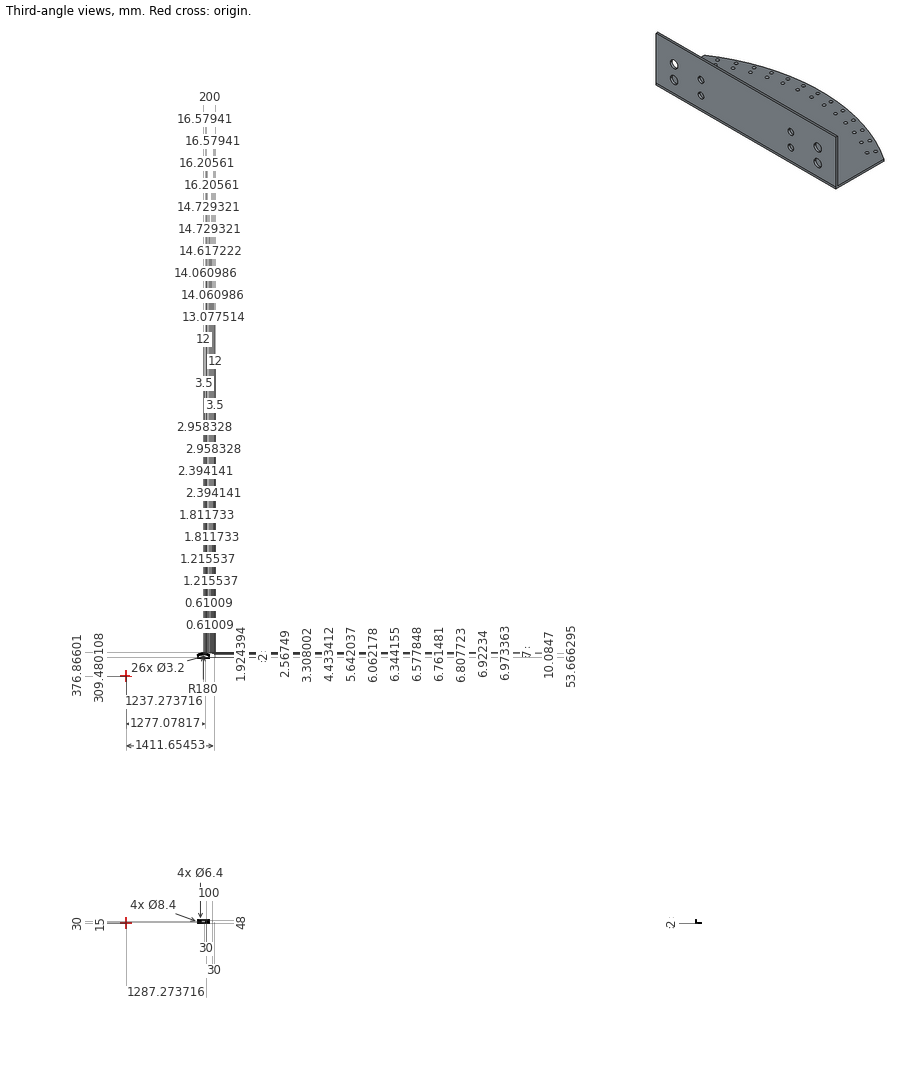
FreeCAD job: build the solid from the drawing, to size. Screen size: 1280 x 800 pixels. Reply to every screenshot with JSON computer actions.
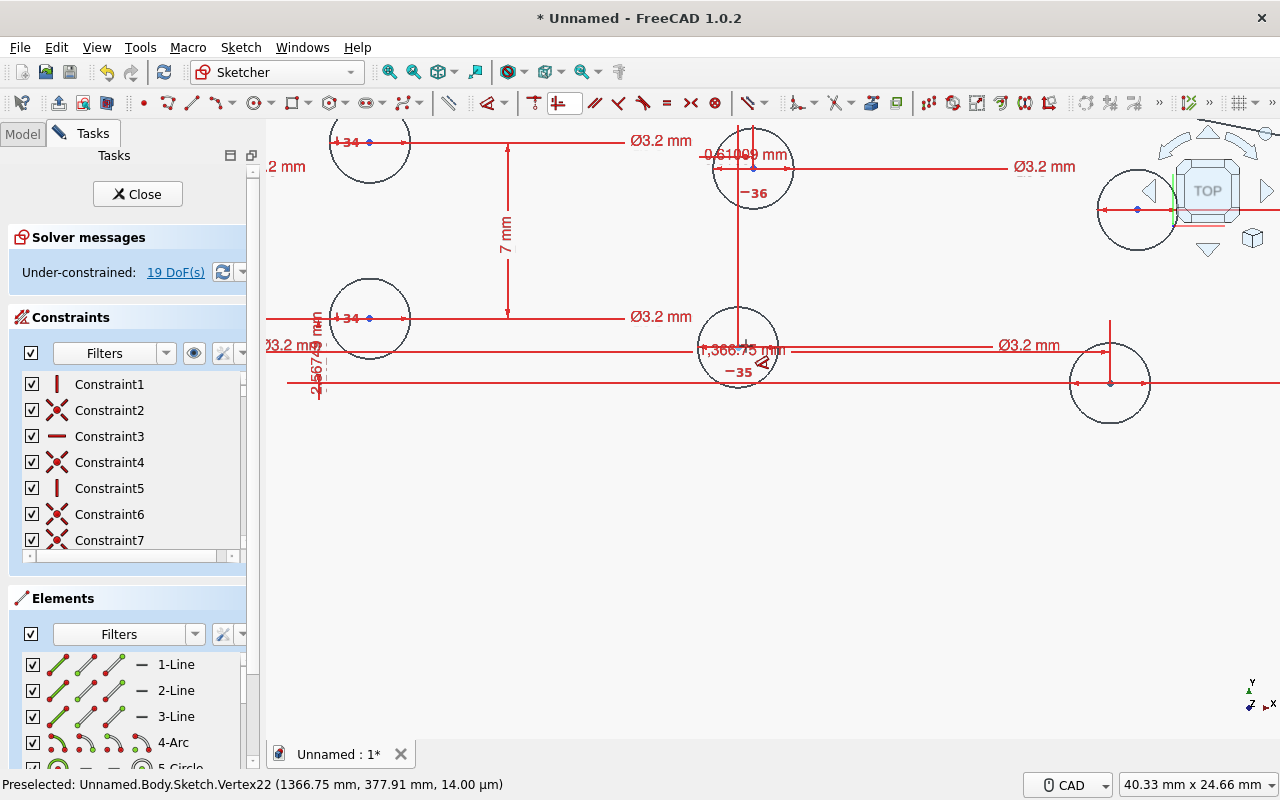
{"action": "left_click", "coordinate": [738, 347]}
{"action": "left_click", "coordinate": [680, 365]}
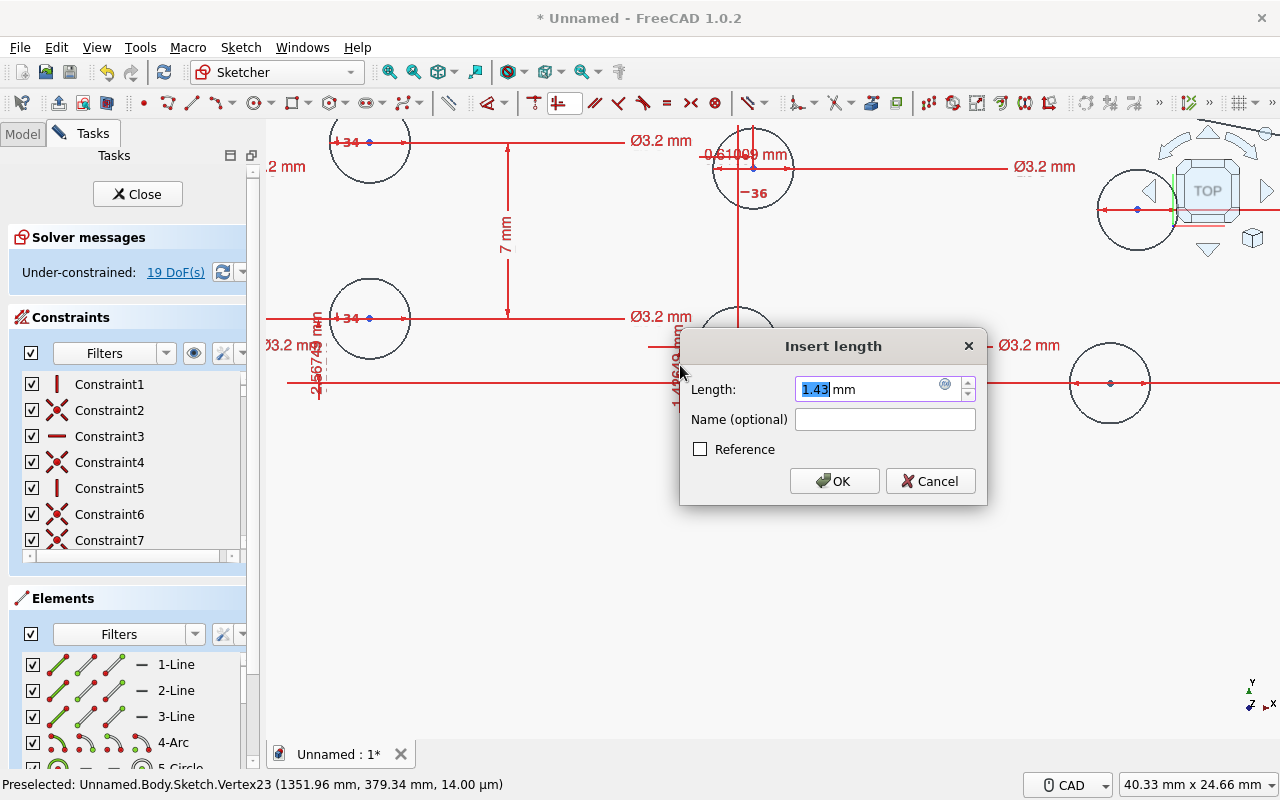
{"action": "type", "text": "1.924394"}
{"action": "key", "text": "Return"}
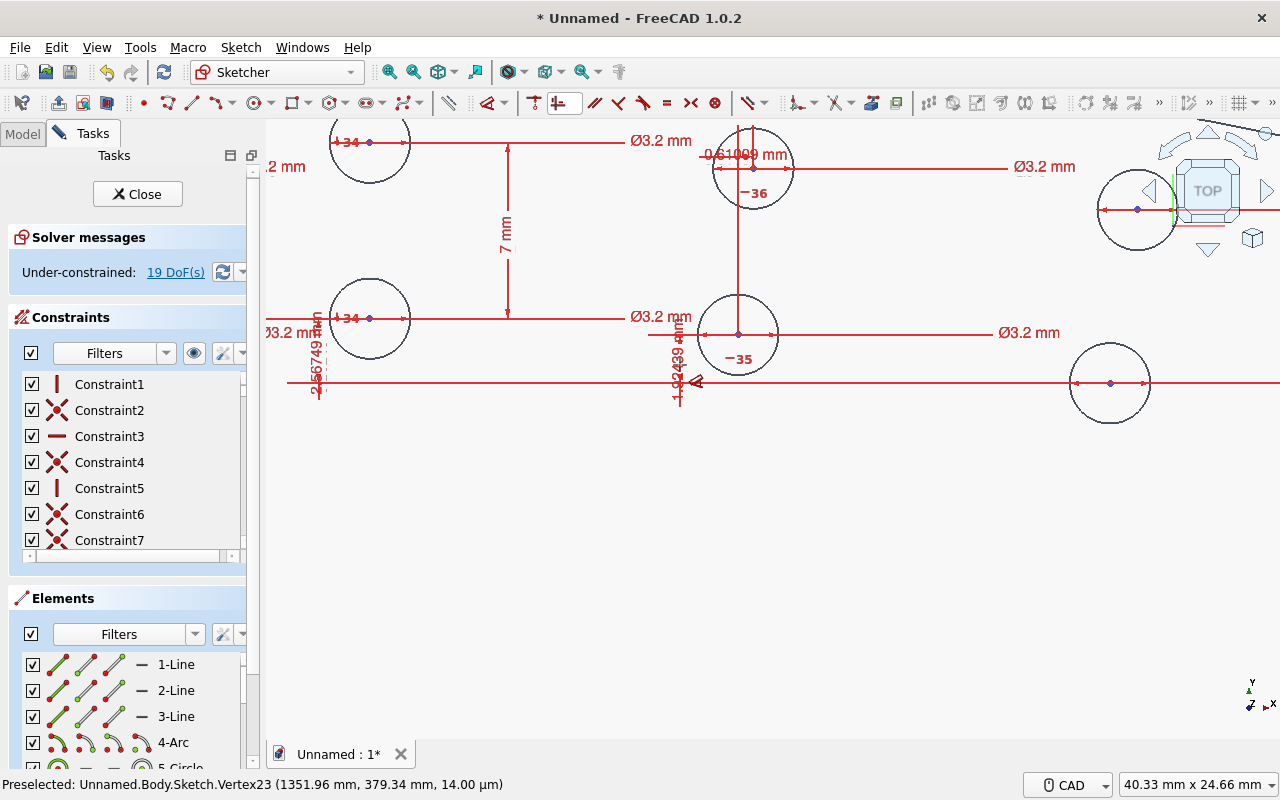
{"action": "scroll", "coordinate": [746, 346], "scroll_direction": "down", "scroll_amount": 11}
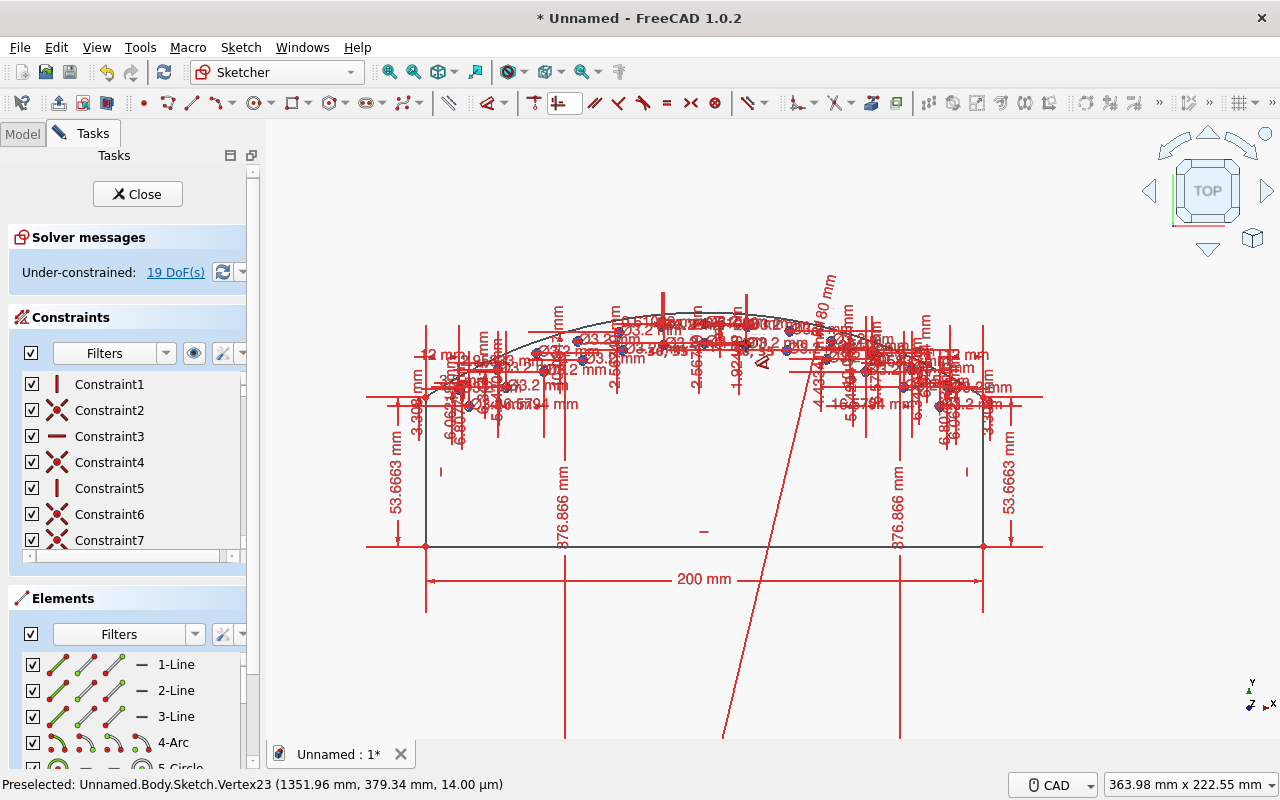
{"action": "scroll", "coordinate": [827, 359], "scroll_direction": "up", "scroll_amount": 11}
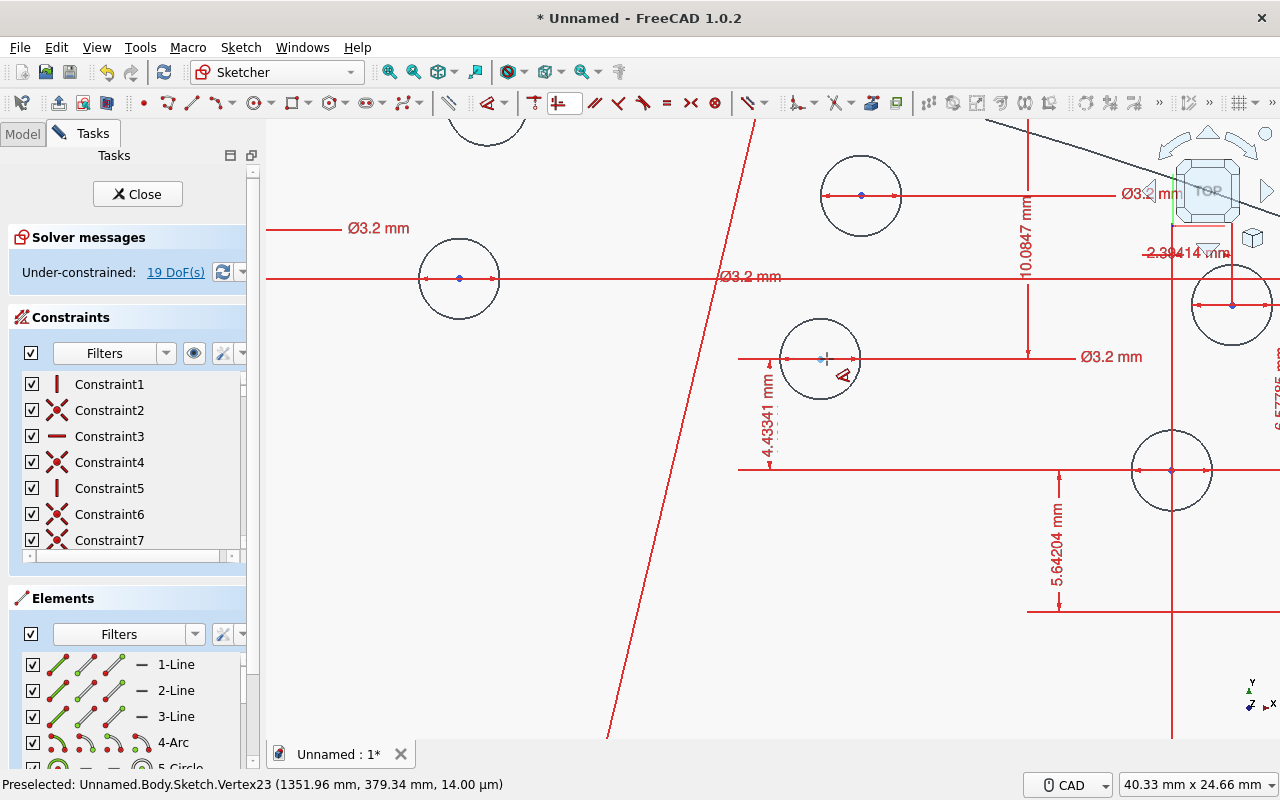
{"action": "left_click", "coordinate": [820, 359]}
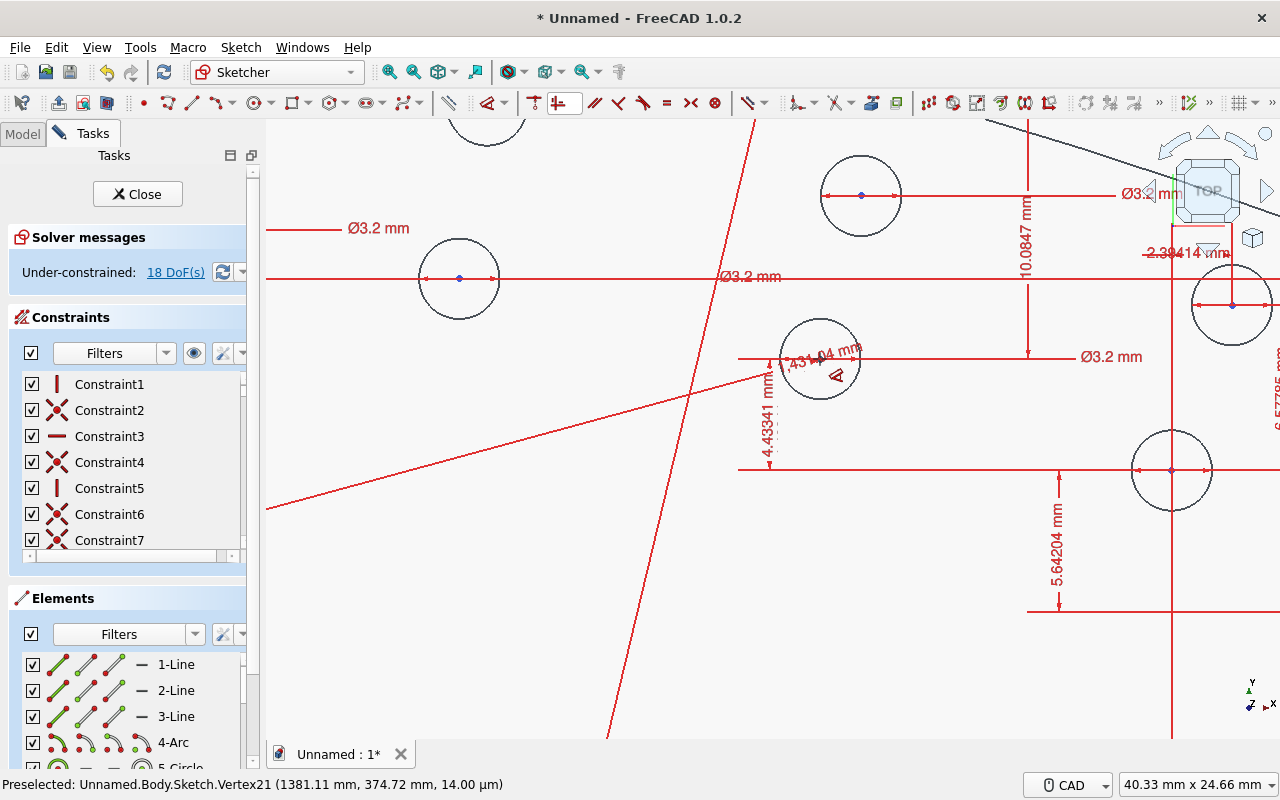
{"action": "left_click", "coordinate": [861, 196]}
{"action": "left_click", "coordinate": [841, 417]}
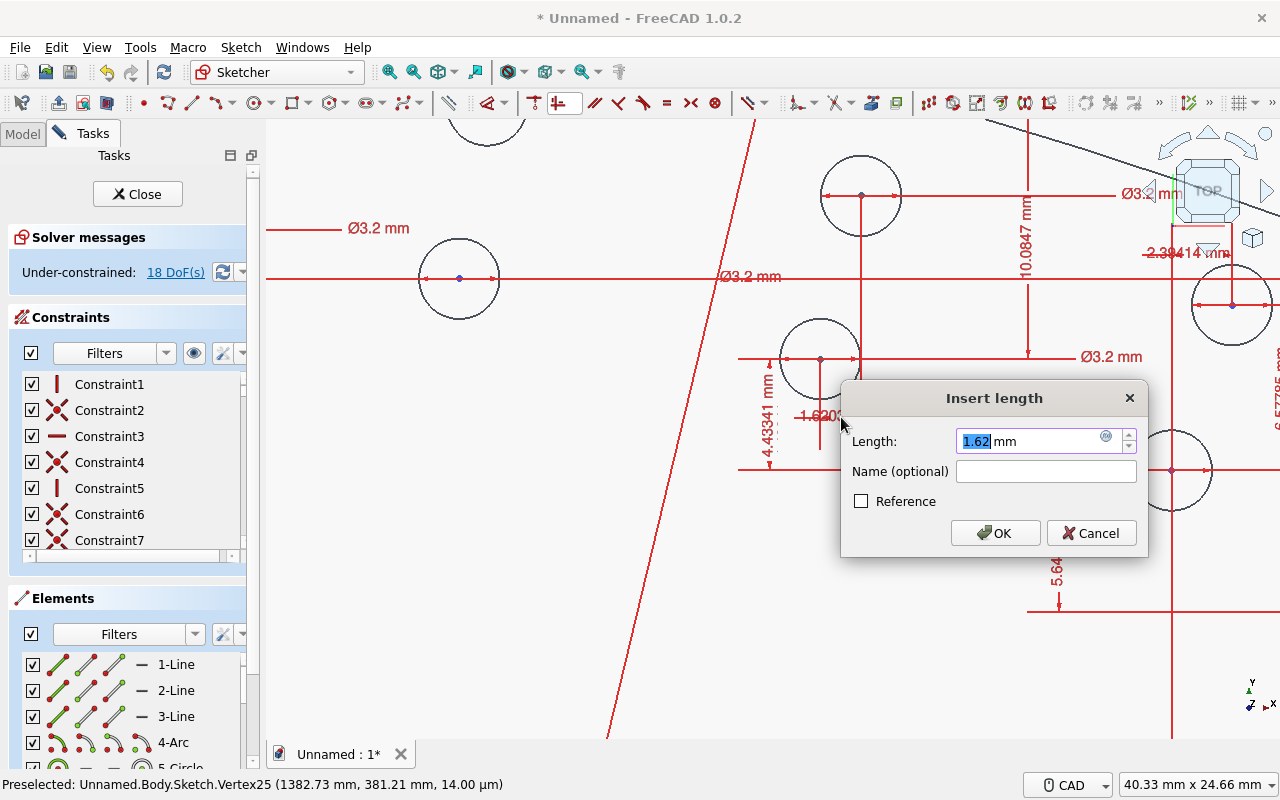
{"action": "type", "text": "1.811733"}
{"action": "key", "text": "Return"}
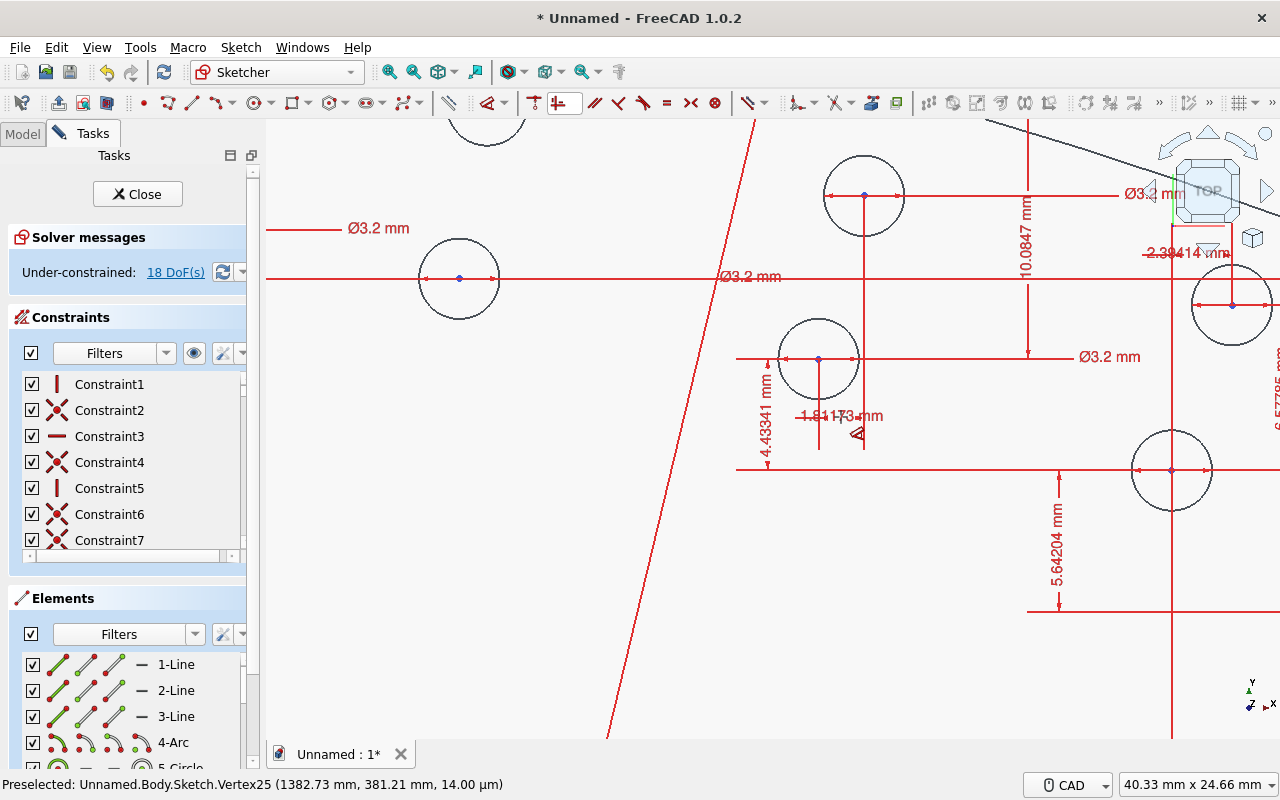
{"action": "scroll", "coordinate": [827, 359], "scroll_direction": "down", "scroll_amount": 11}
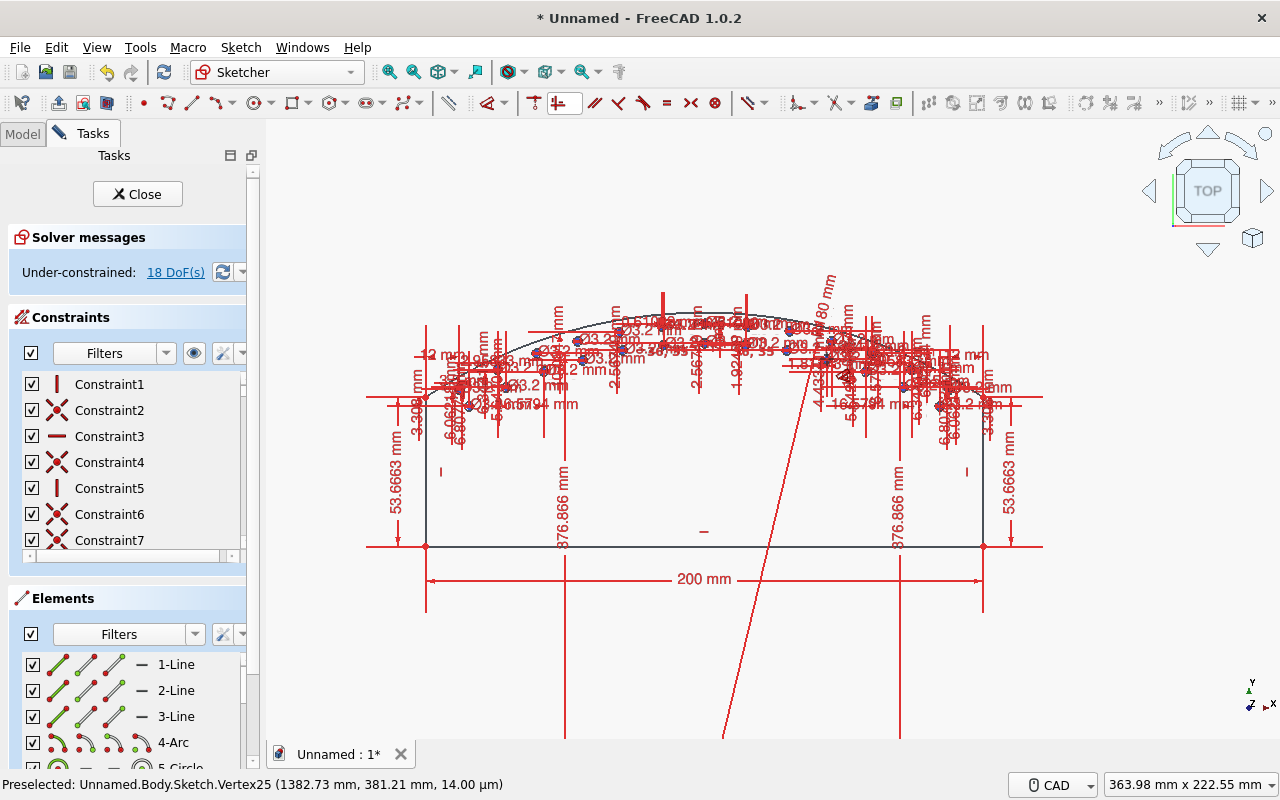
{"action": "left_click", "coordinate": [787, 350]}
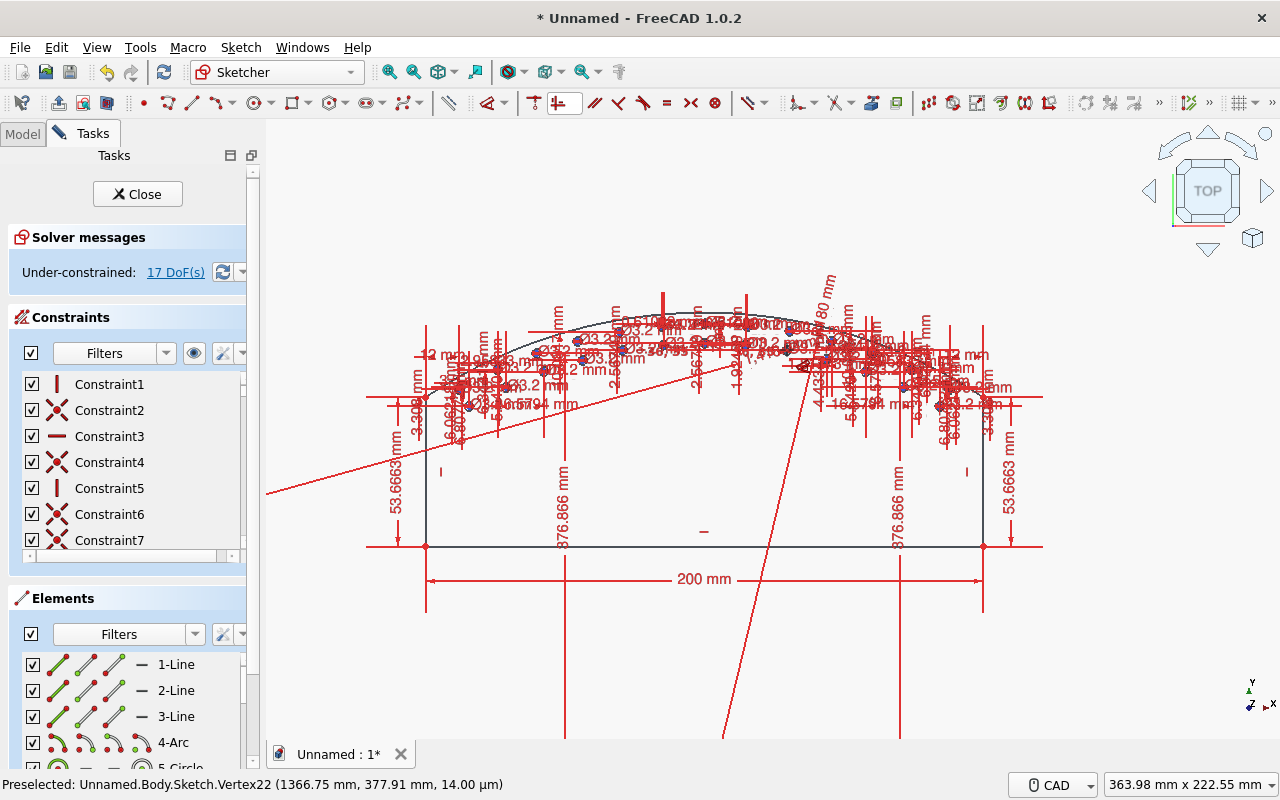
{"action": "left_click", "coordinate": [832, 341]}
{"action": "left_click", "coordinate": [809, 283]}